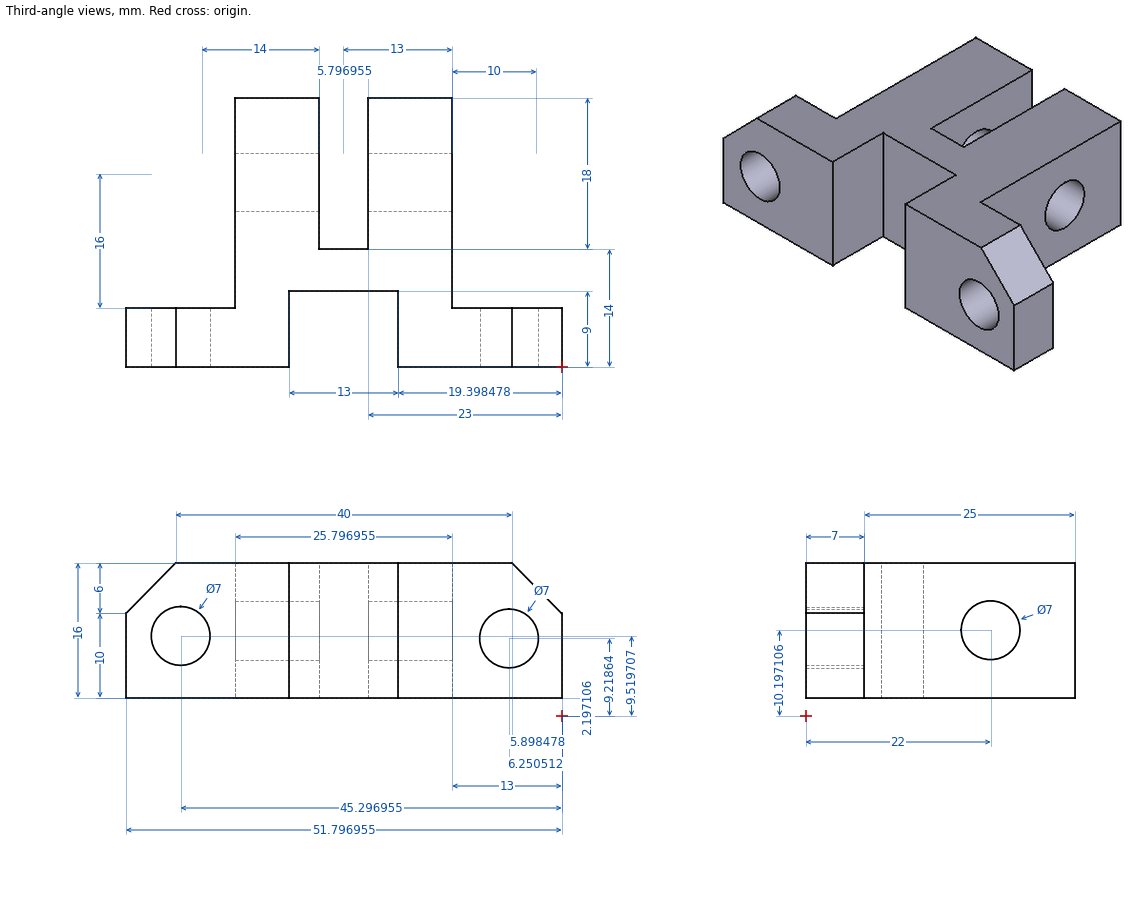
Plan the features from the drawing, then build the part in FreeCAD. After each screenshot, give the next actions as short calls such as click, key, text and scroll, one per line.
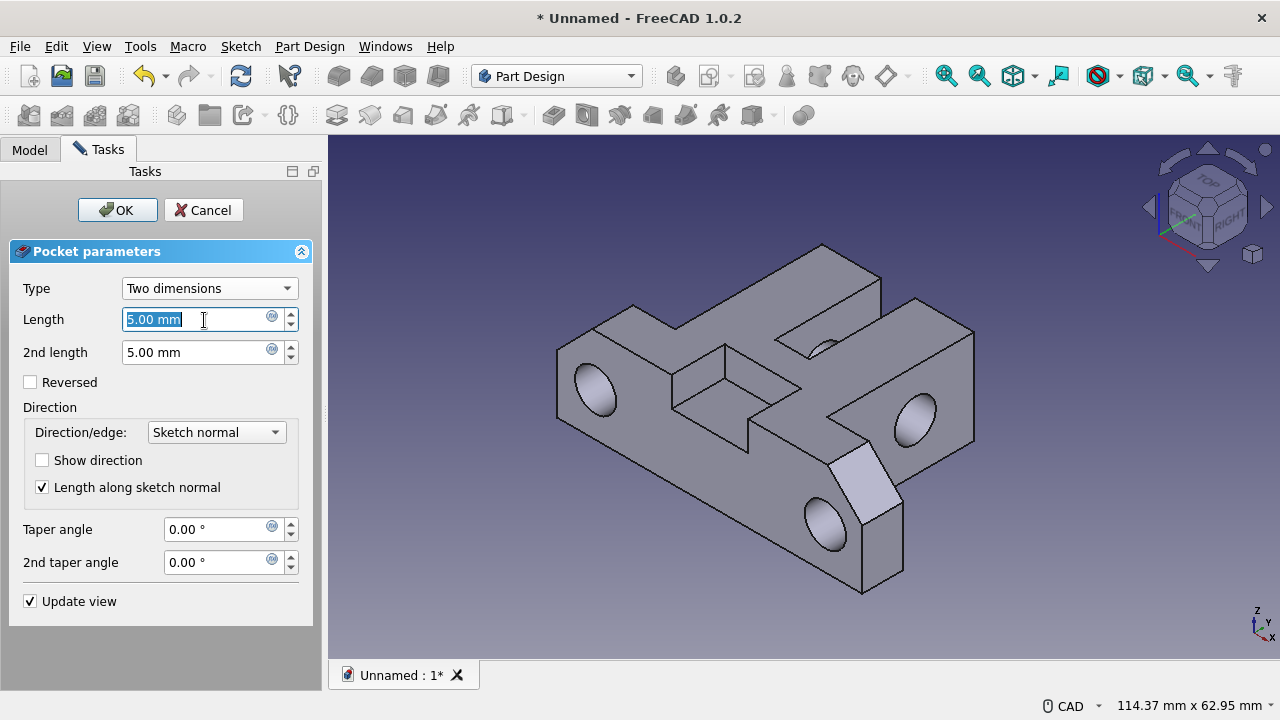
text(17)
key(Tab)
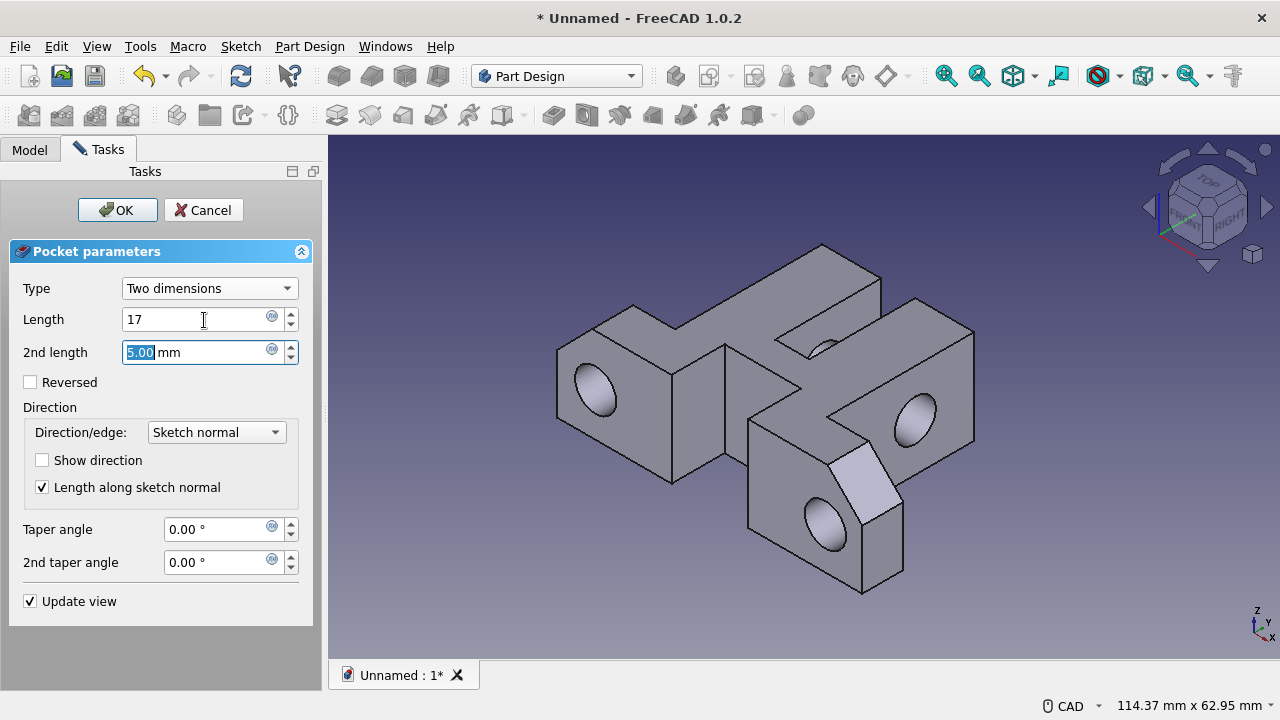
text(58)
key(Tab)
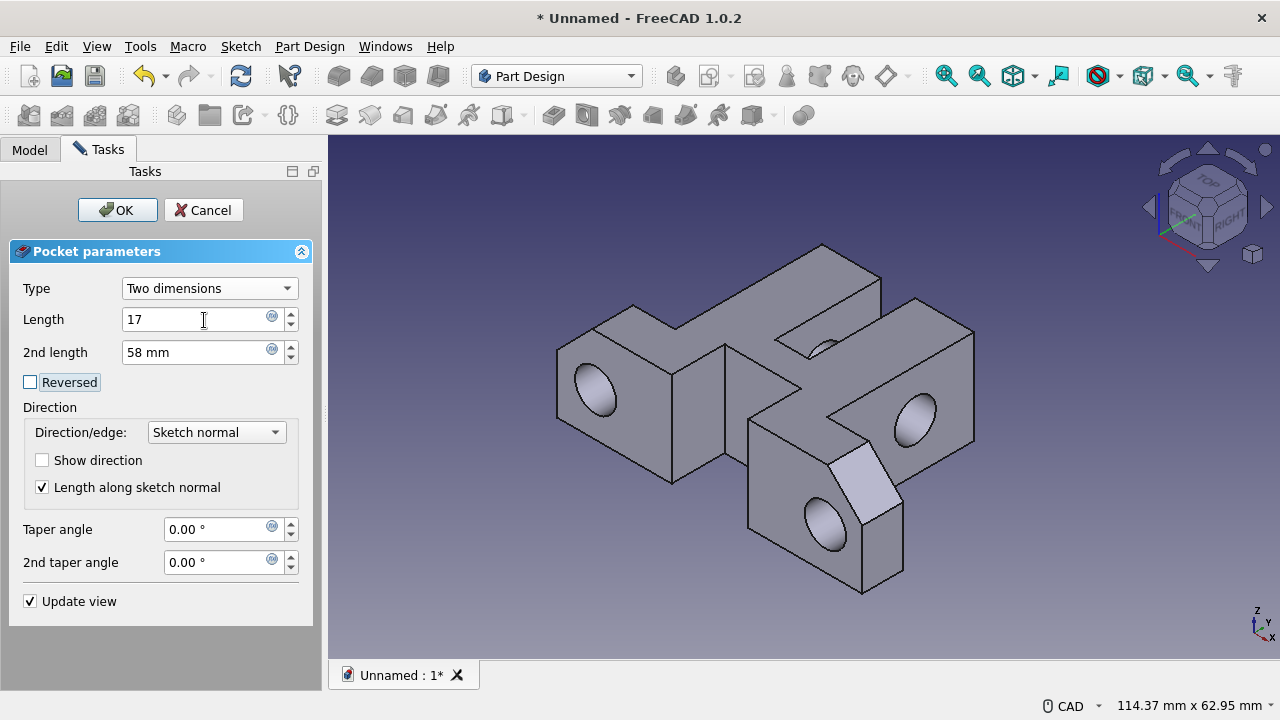
click(31, 382)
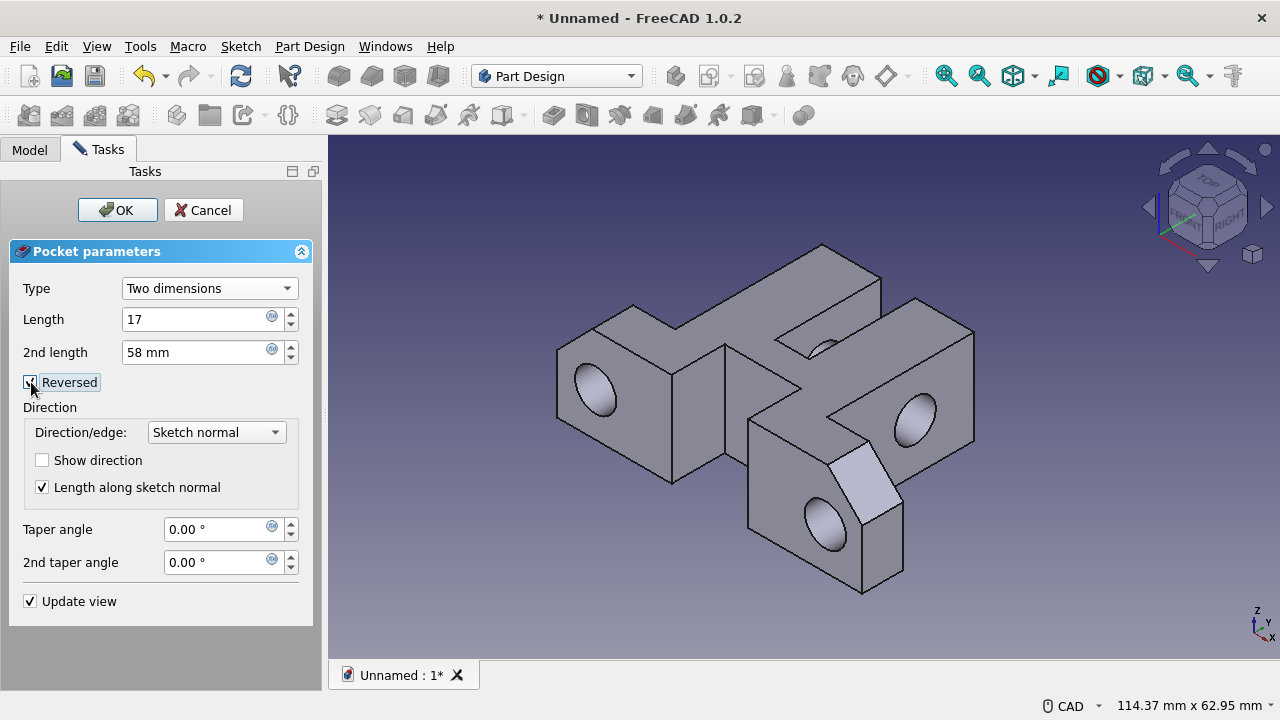
click(118, 210)